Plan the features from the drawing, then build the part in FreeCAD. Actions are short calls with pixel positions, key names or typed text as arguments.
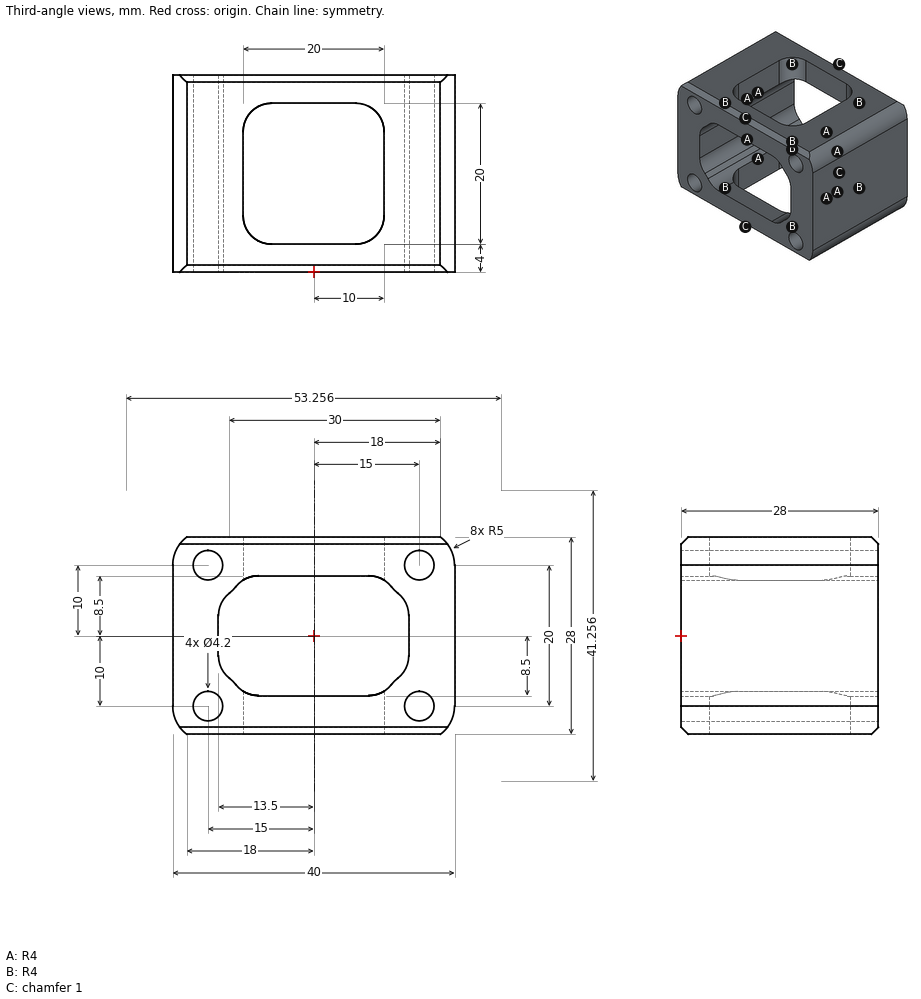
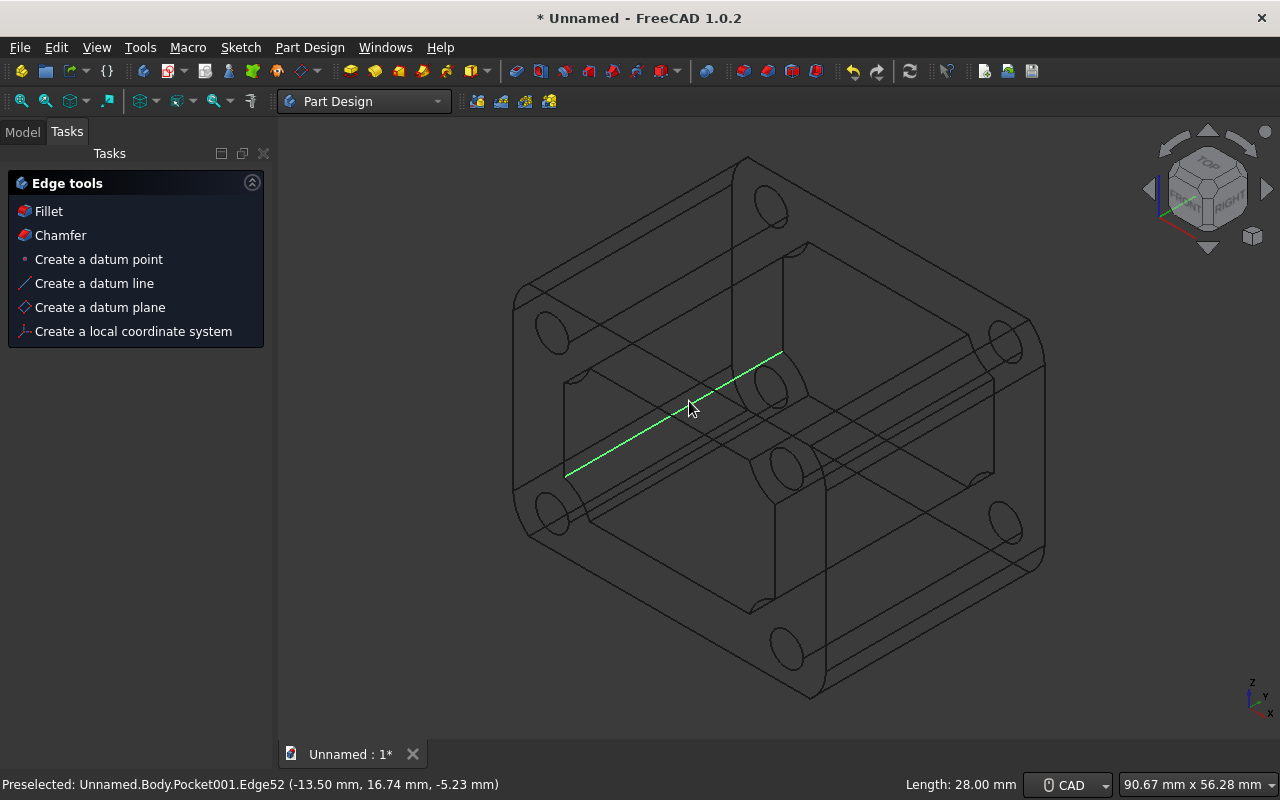
click(699, 458, ctrl)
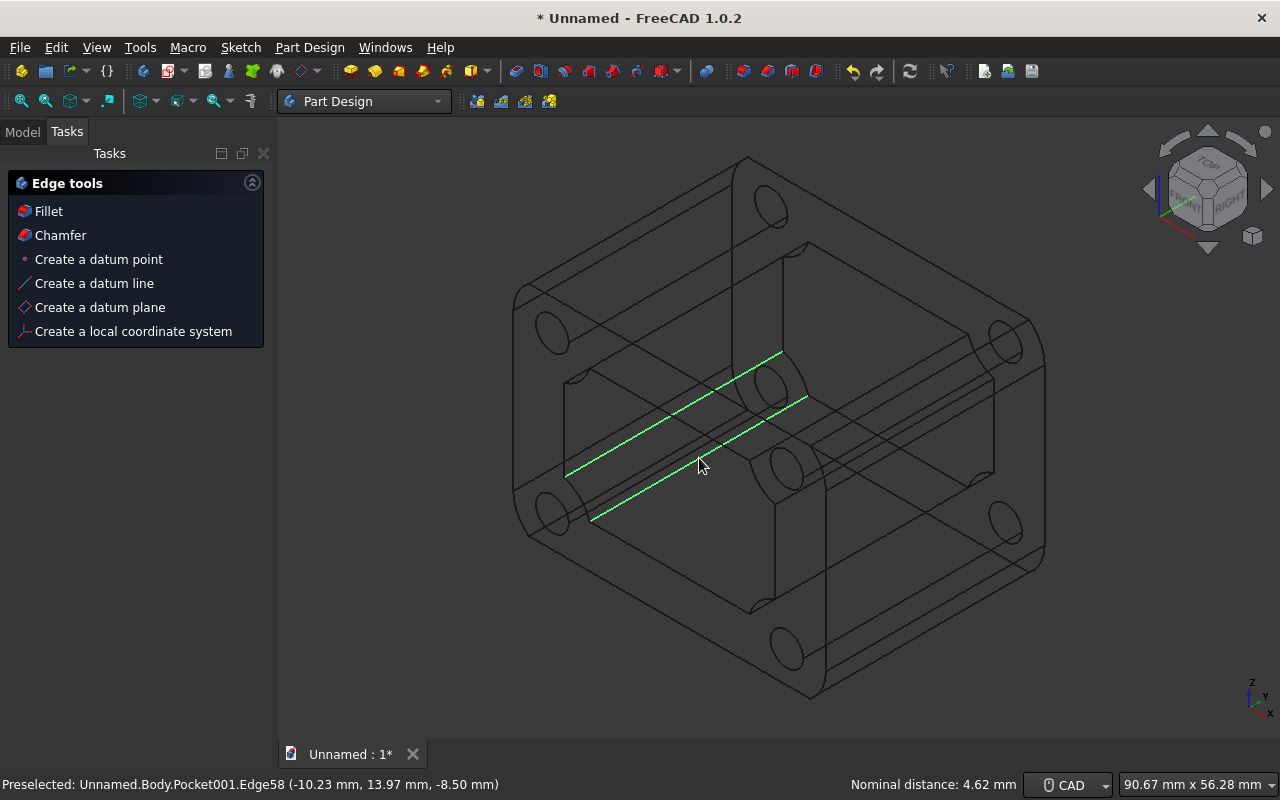
click(884, 535, ctrl)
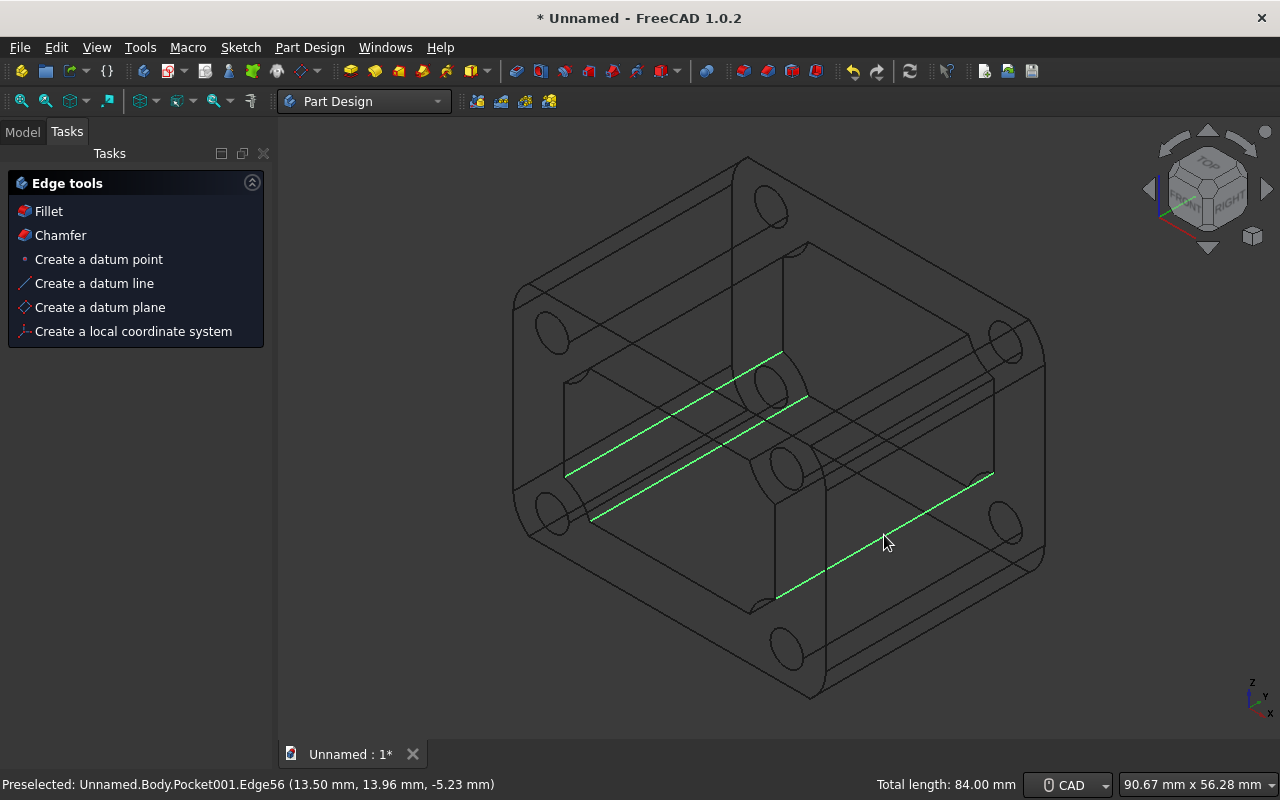
click(884, 441, ctrl)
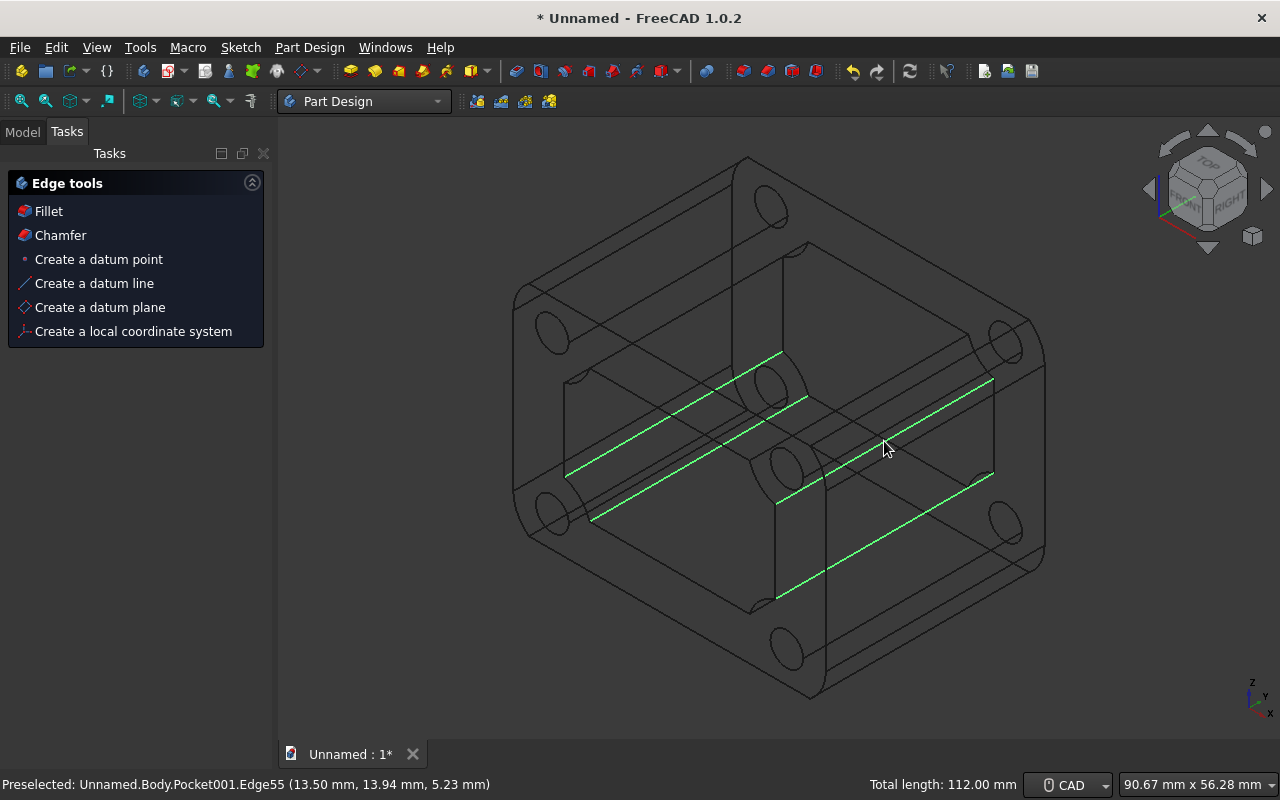
click(859, 396, ctrl)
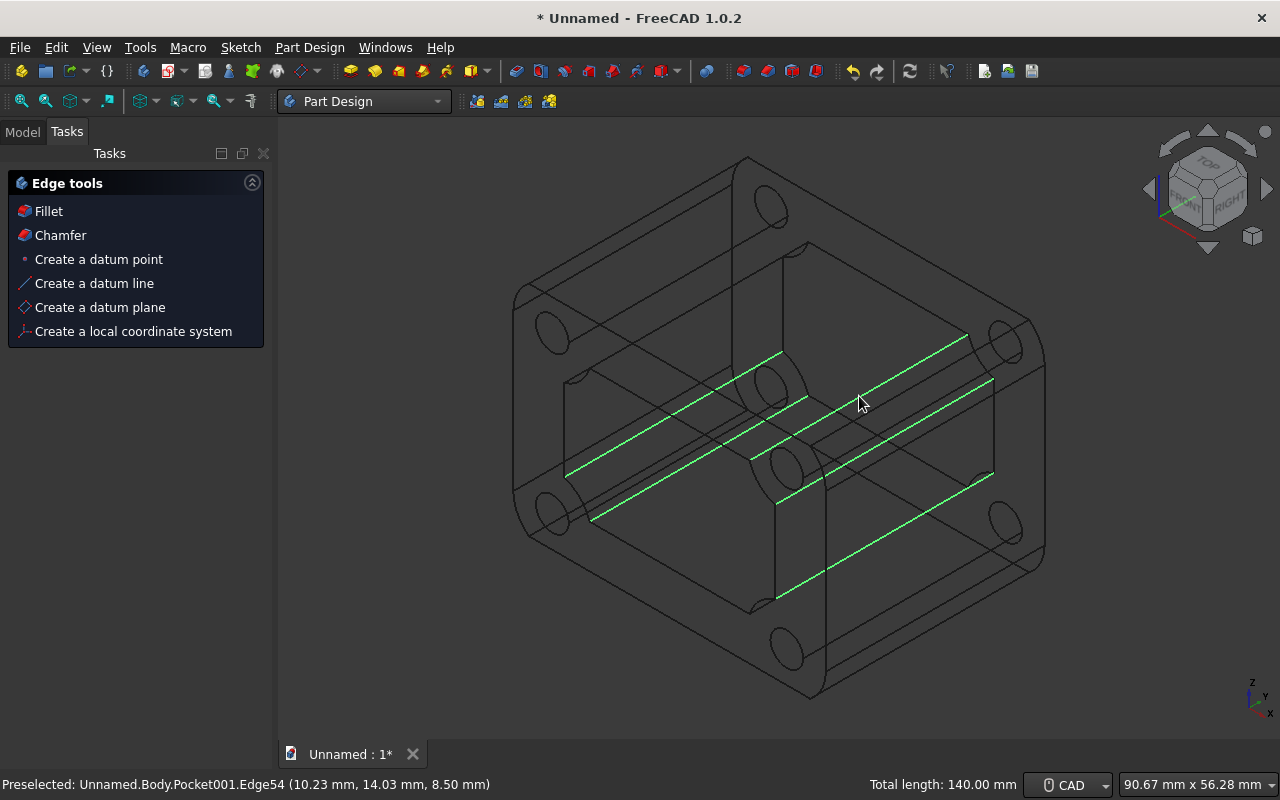
click(699, 304, ctrl)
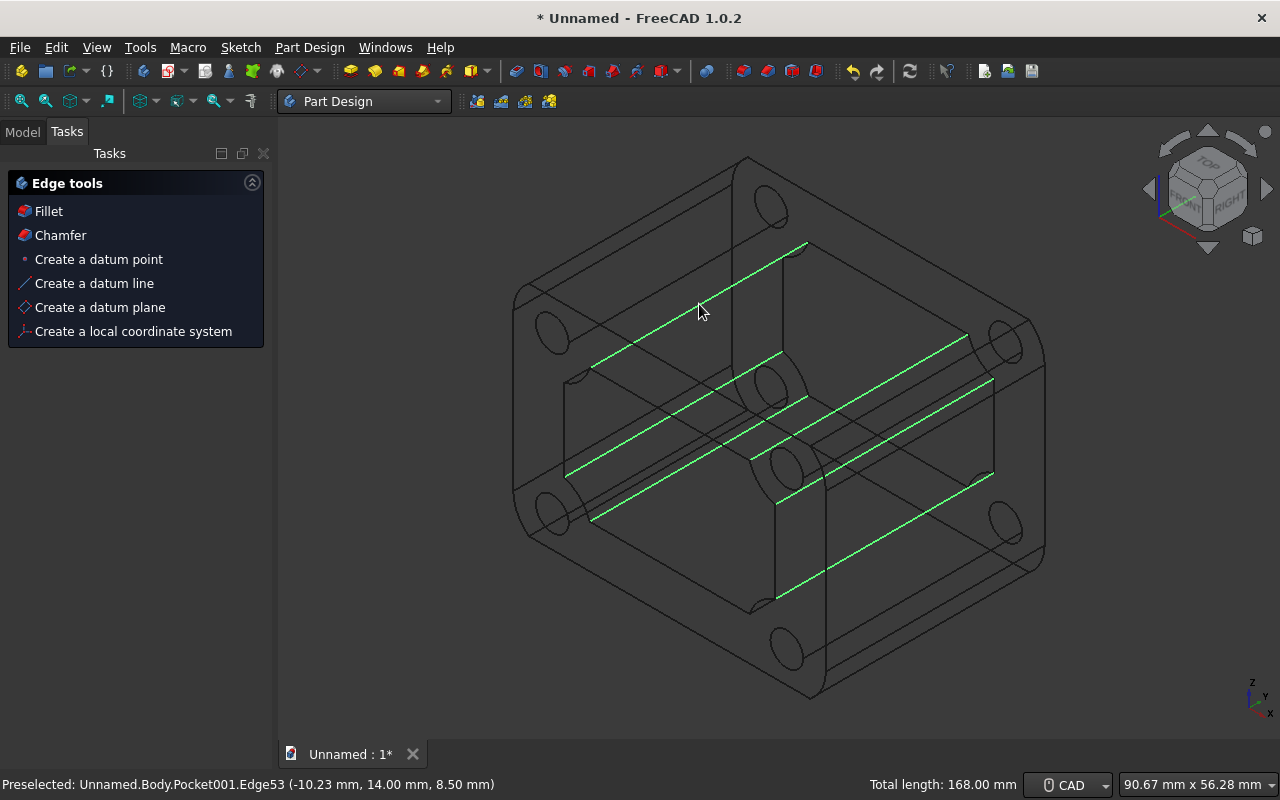
key(2)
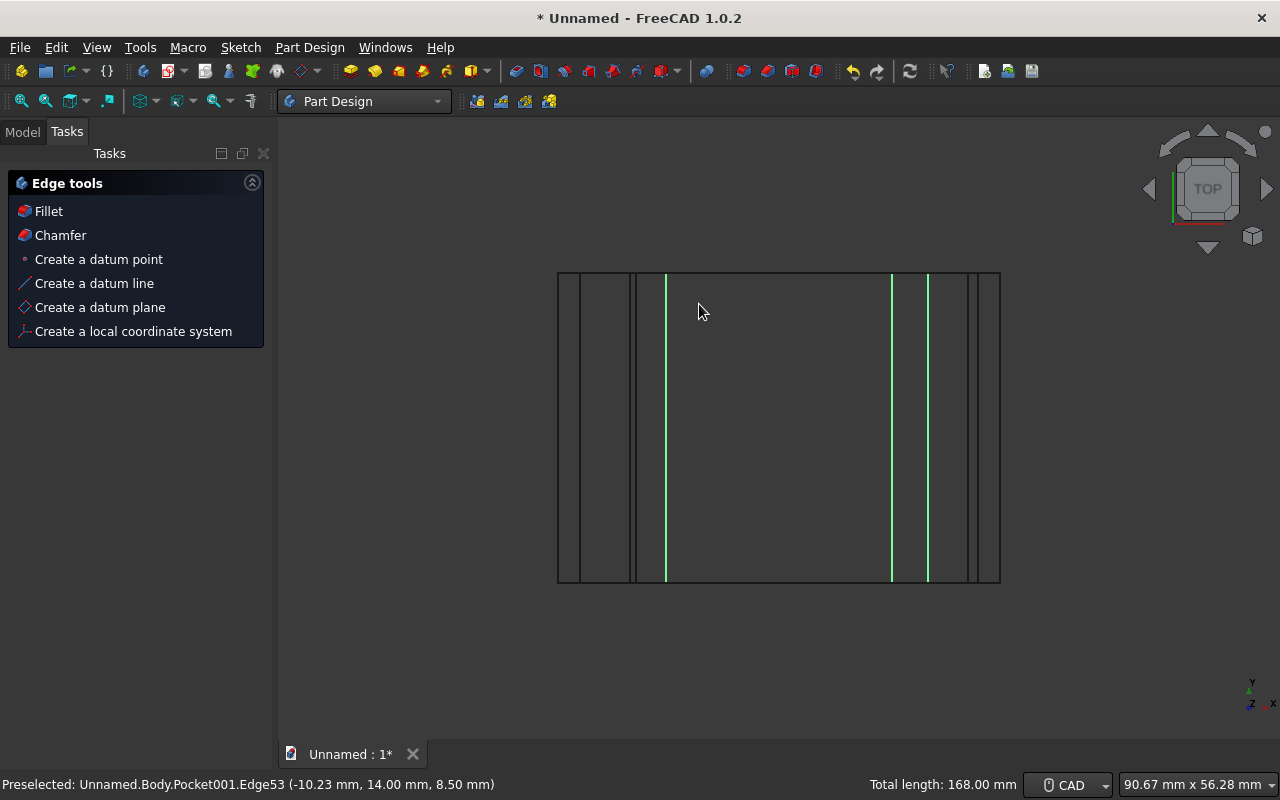
click(630, 427, ctrl)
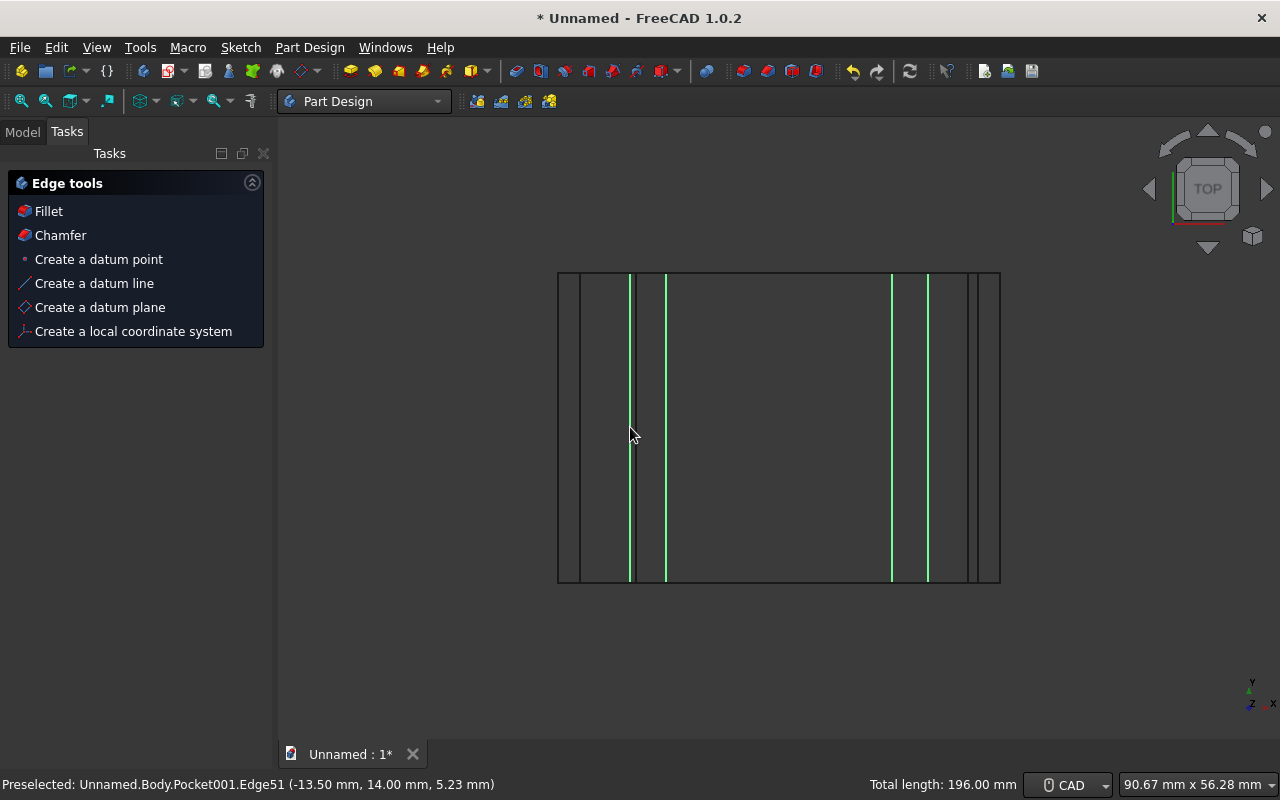
key(1)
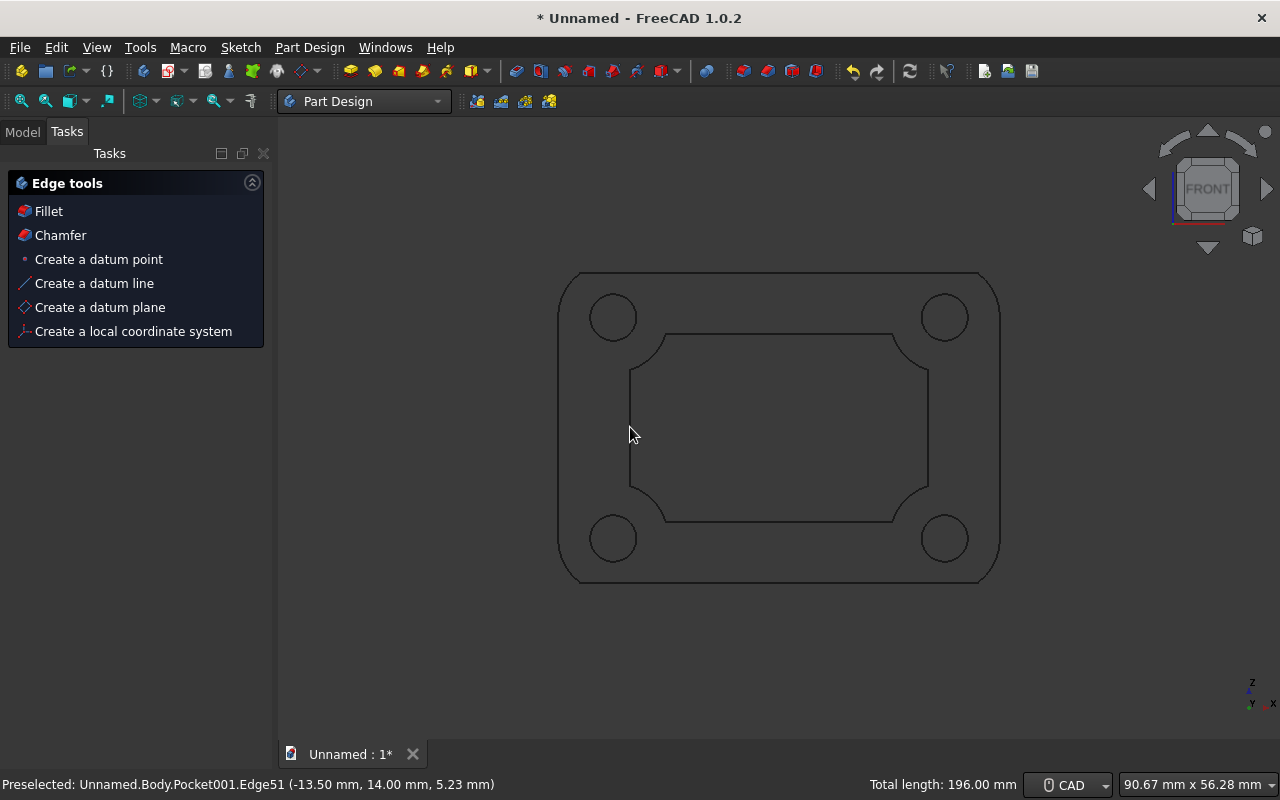
key(3)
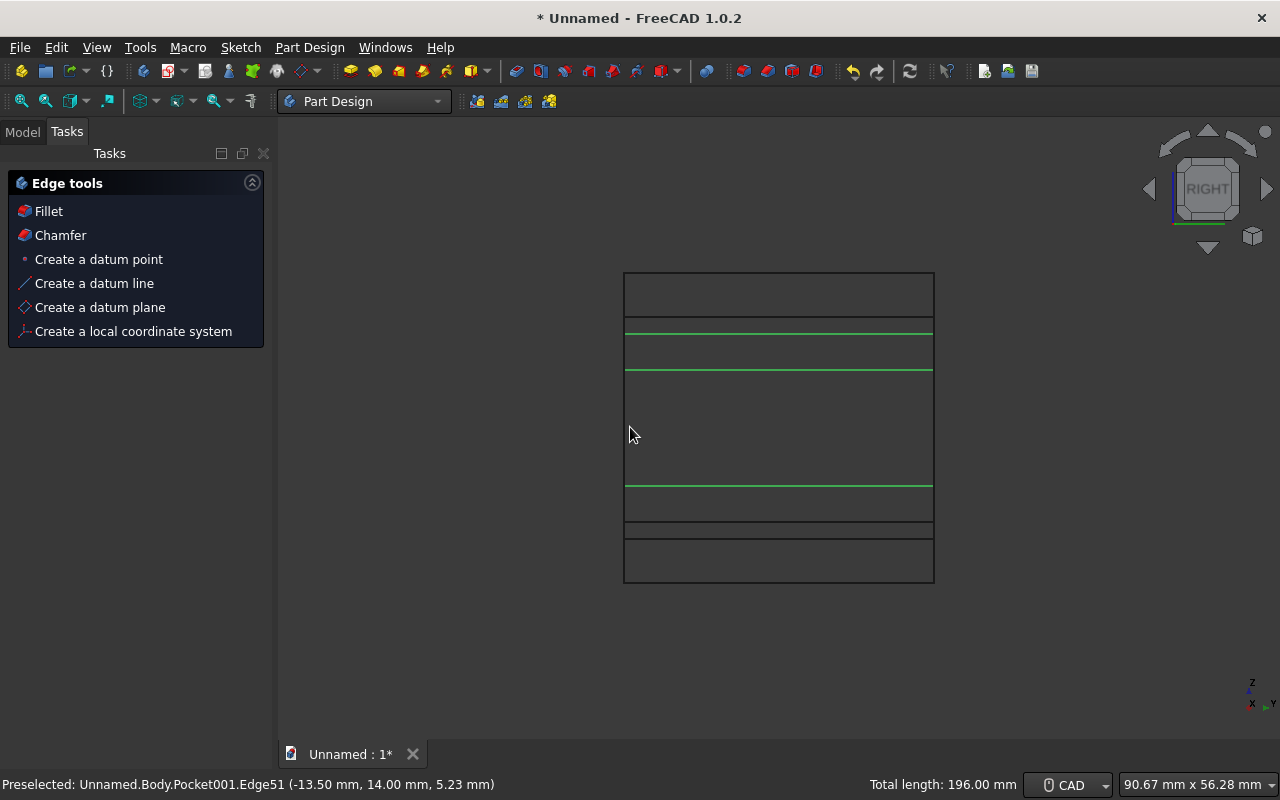
click(779, 521, ctrl)